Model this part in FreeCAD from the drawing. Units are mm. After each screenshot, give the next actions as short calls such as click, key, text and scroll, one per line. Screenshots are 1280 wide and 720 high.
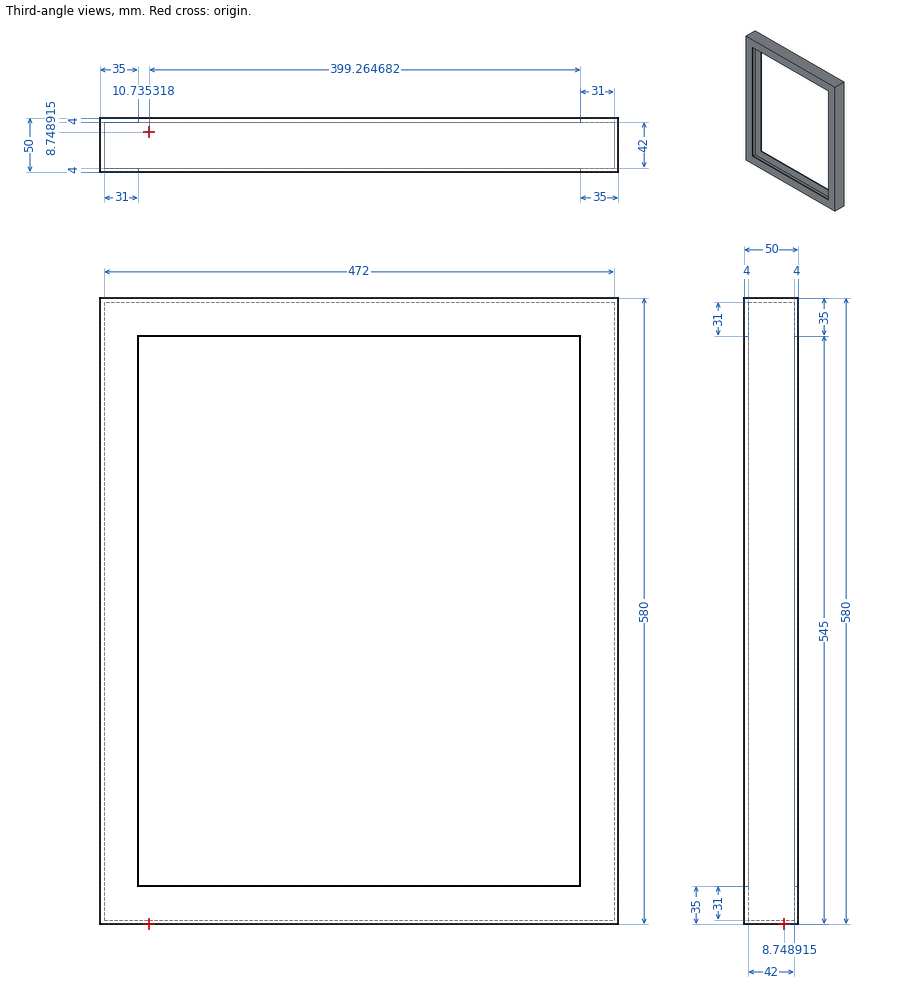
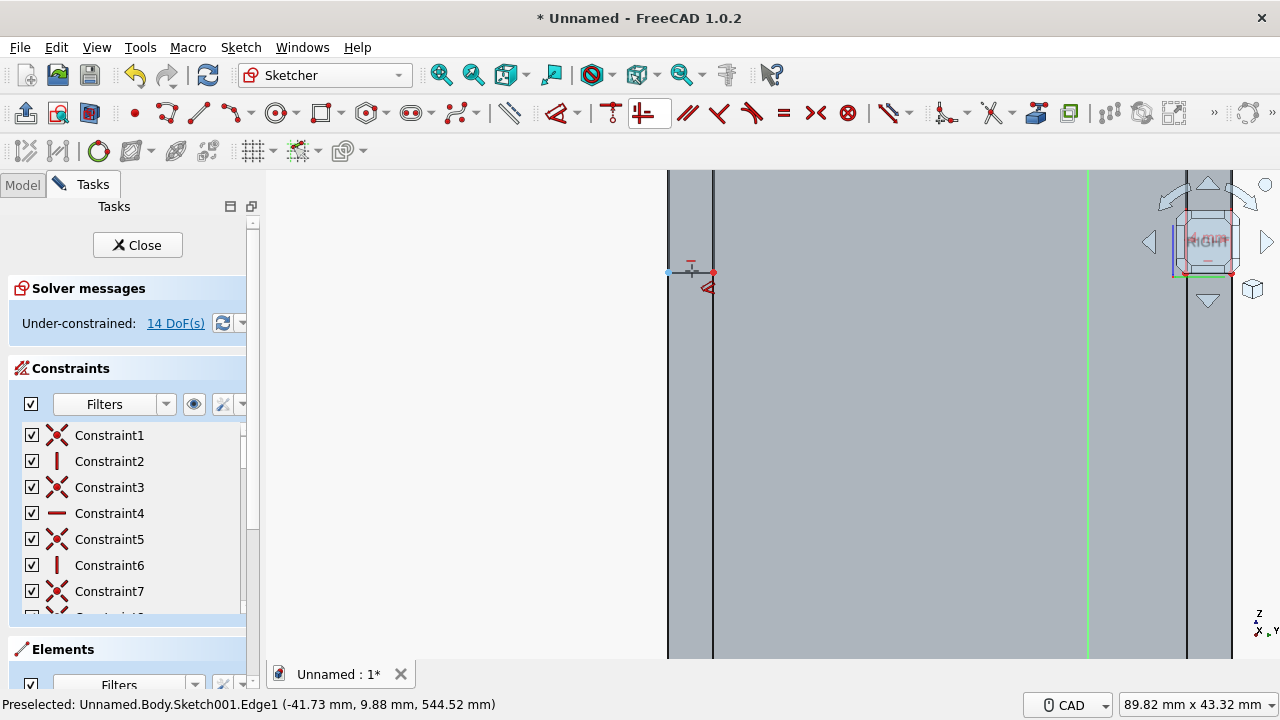
click(682, 273)
click(691, 239)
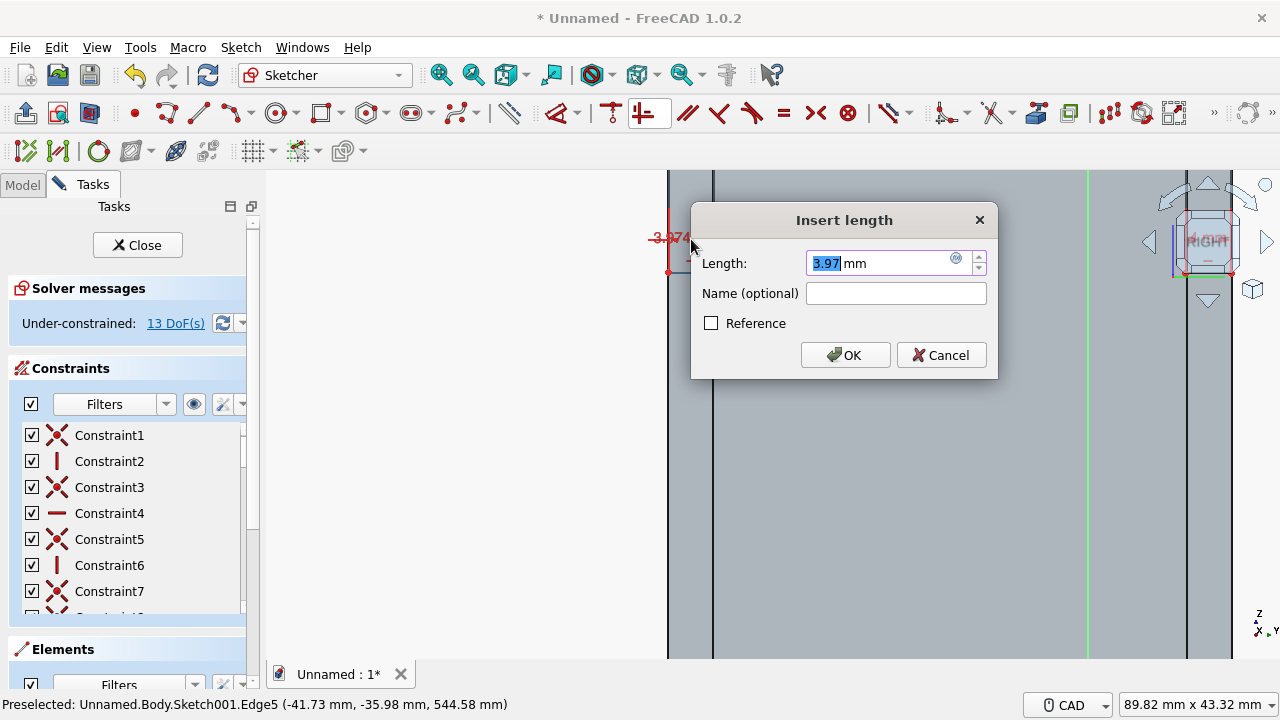
text(4)
key(Return)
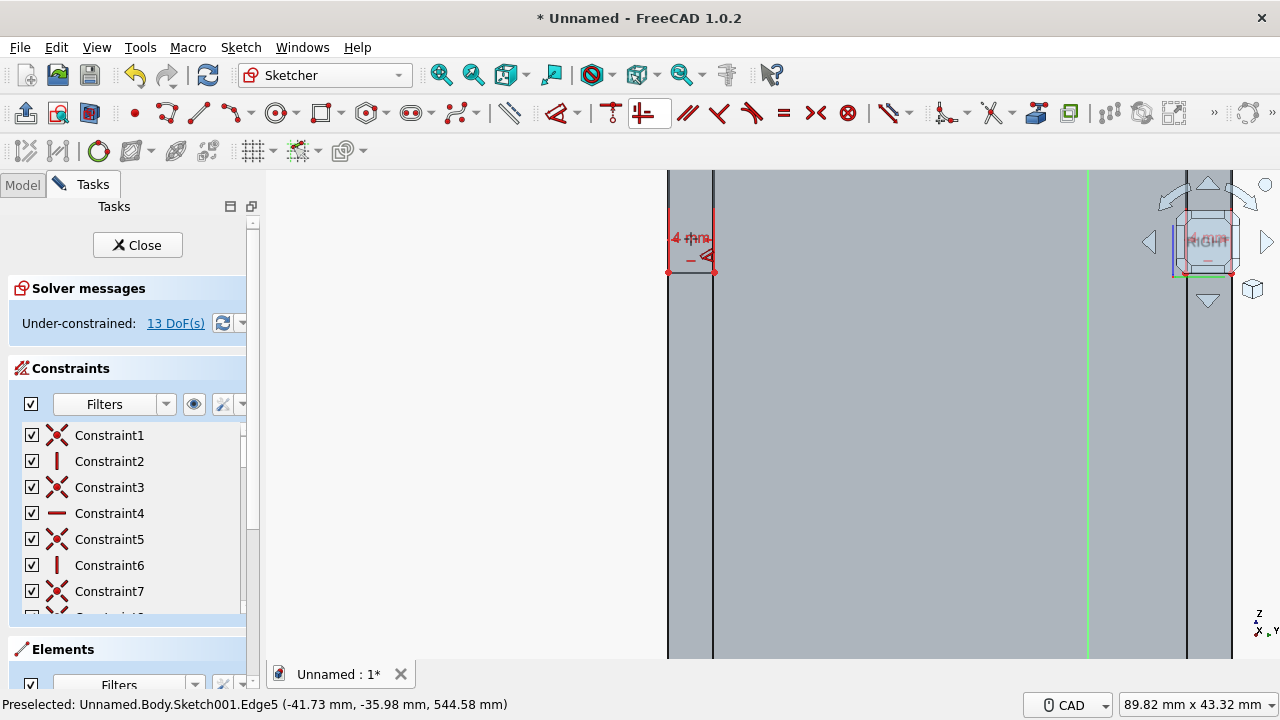
scroll(692, 271, down, 15)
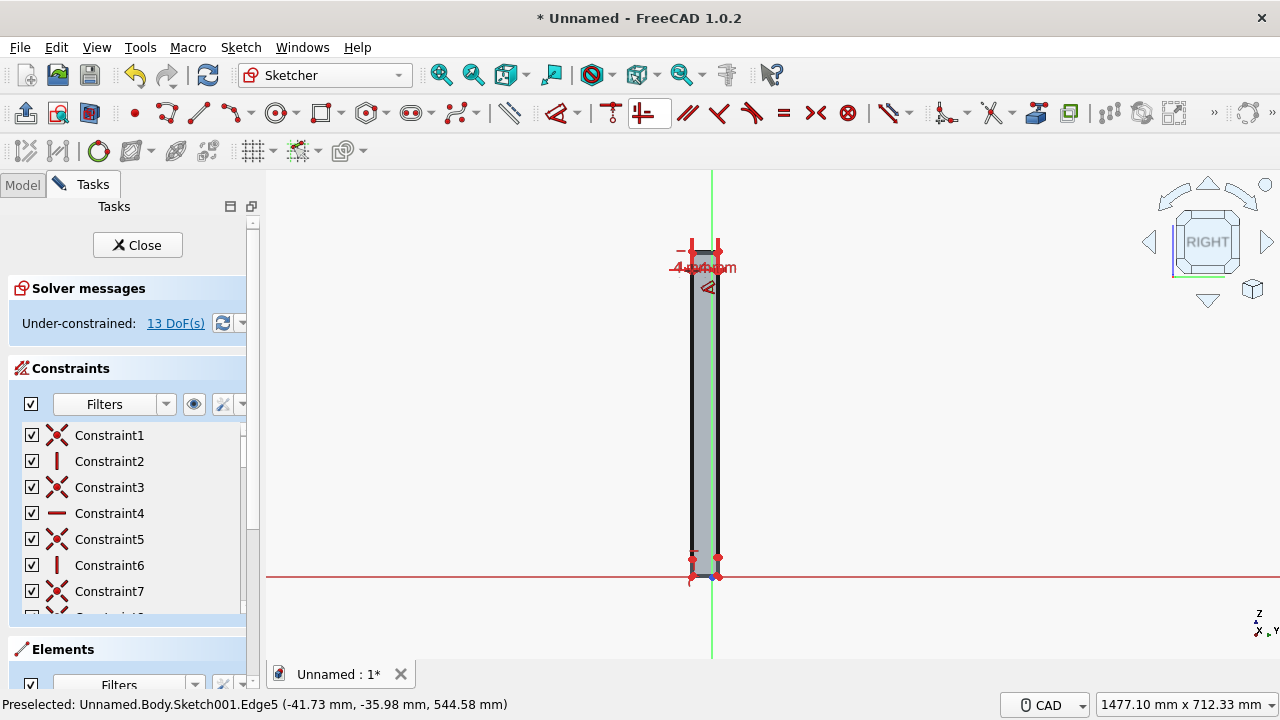
scroll(693, 559, up, 15)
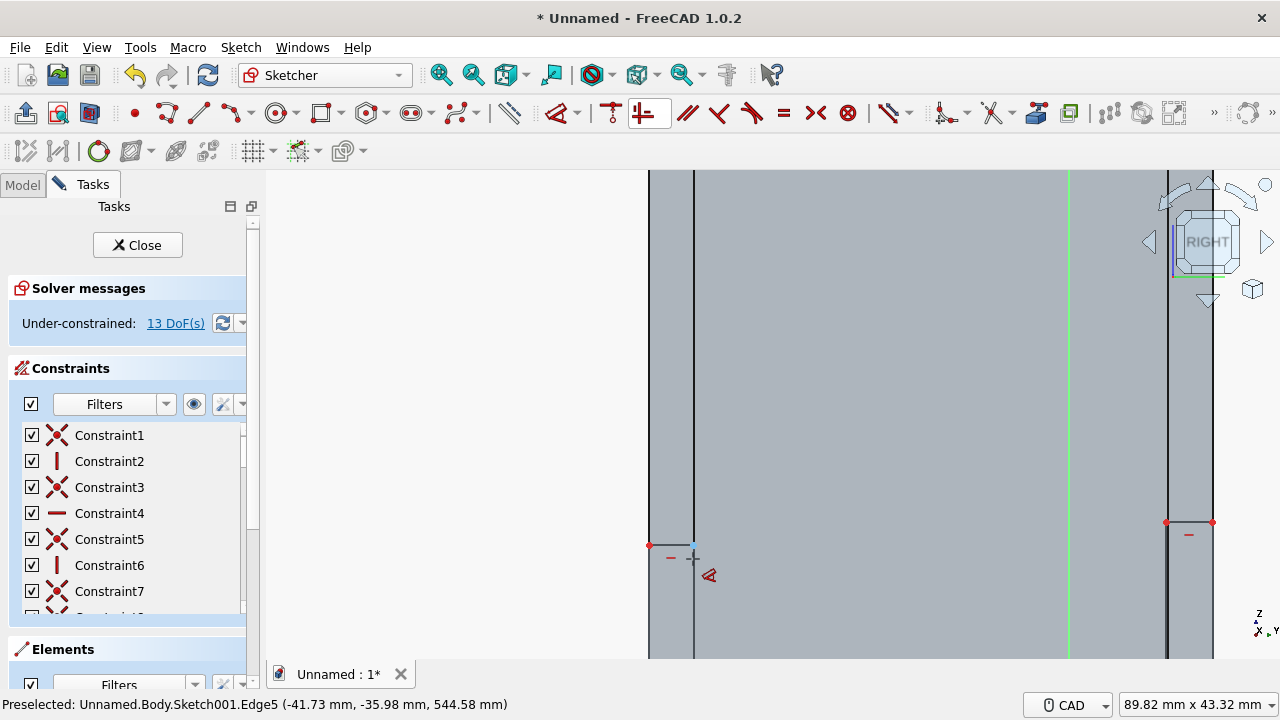
click(680, 545)
click(671, 579)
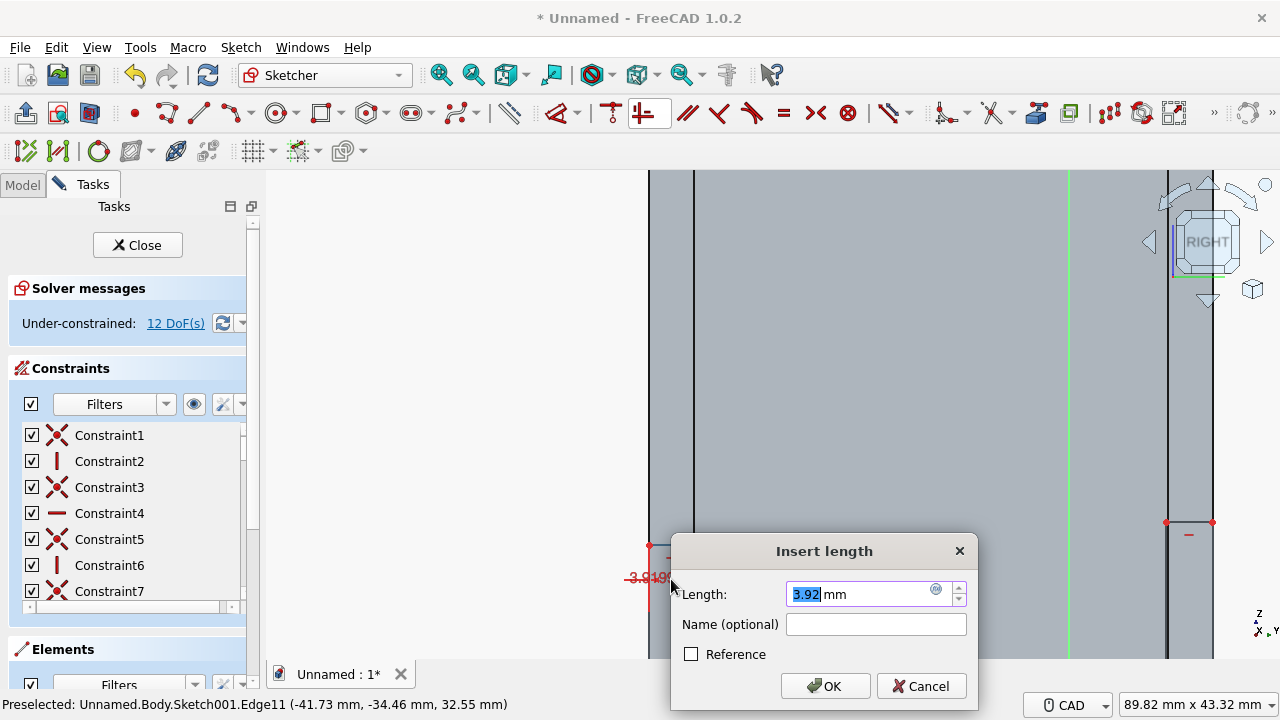
text(4)
key(Return)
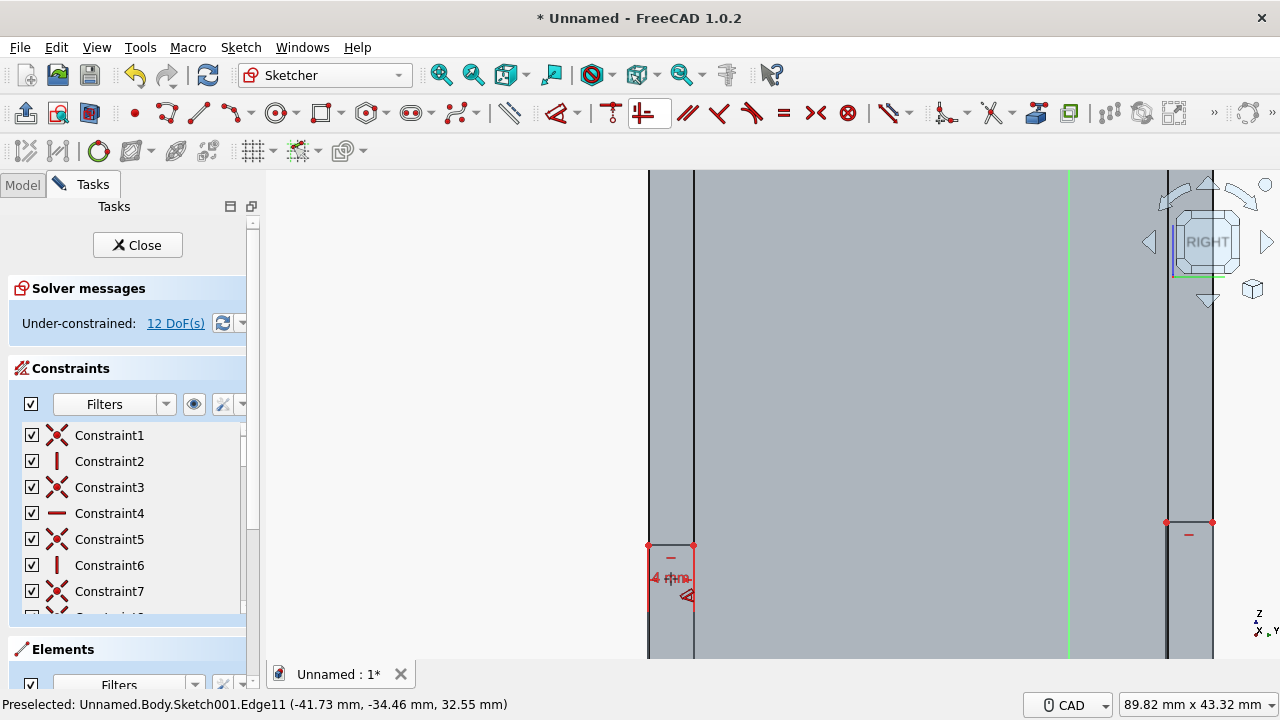
scroll(693, 560, down, 15)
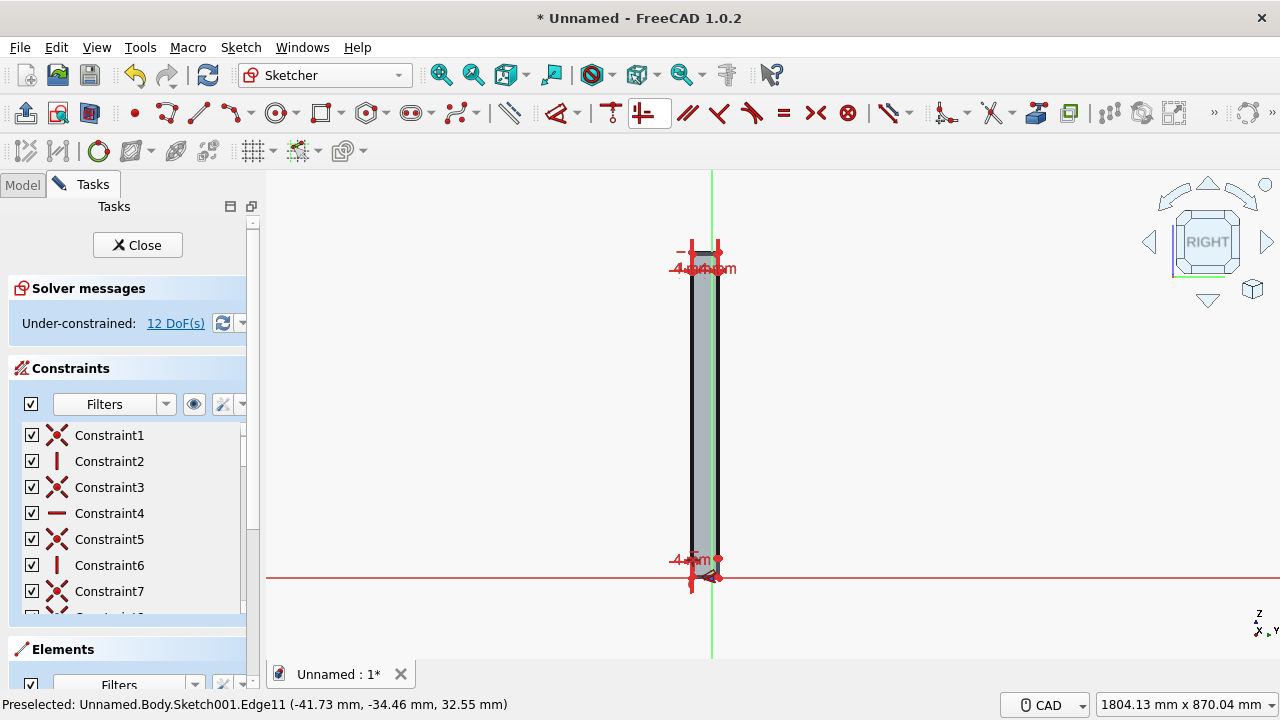
scroll(719, 559, up, 15)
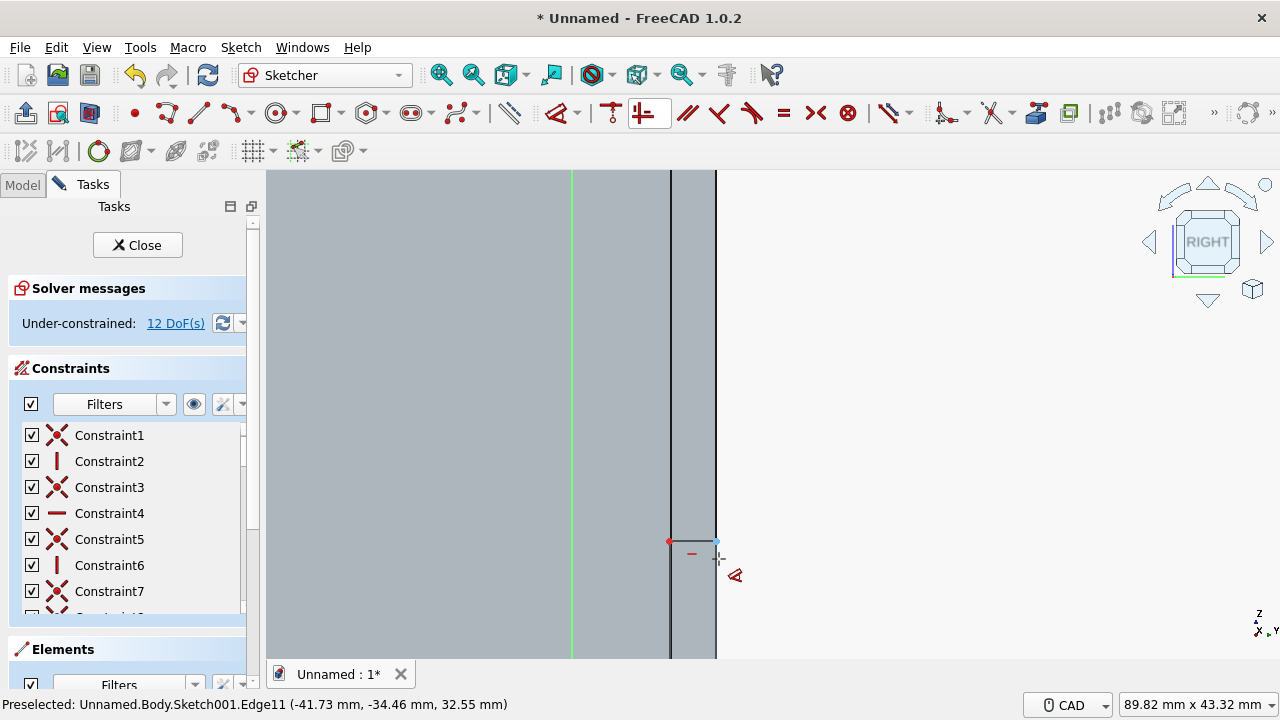
click(702, 541)
click(693, 575)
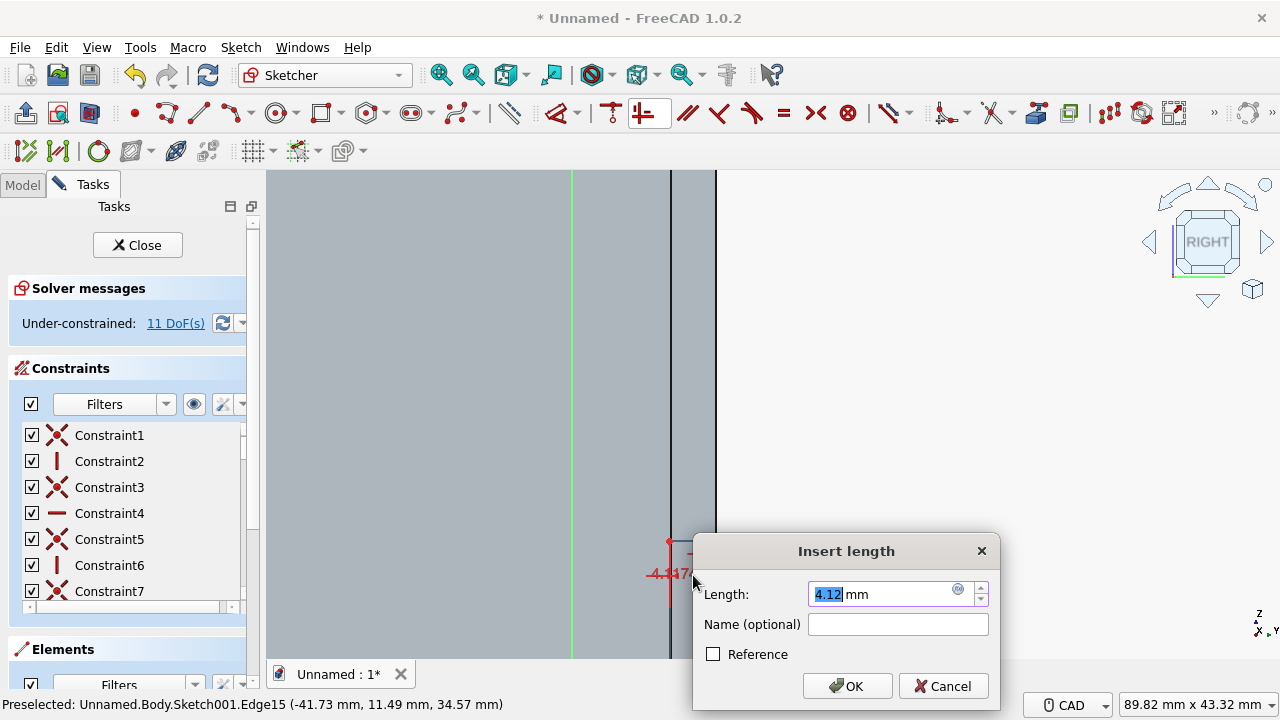
text(4)
key(Return)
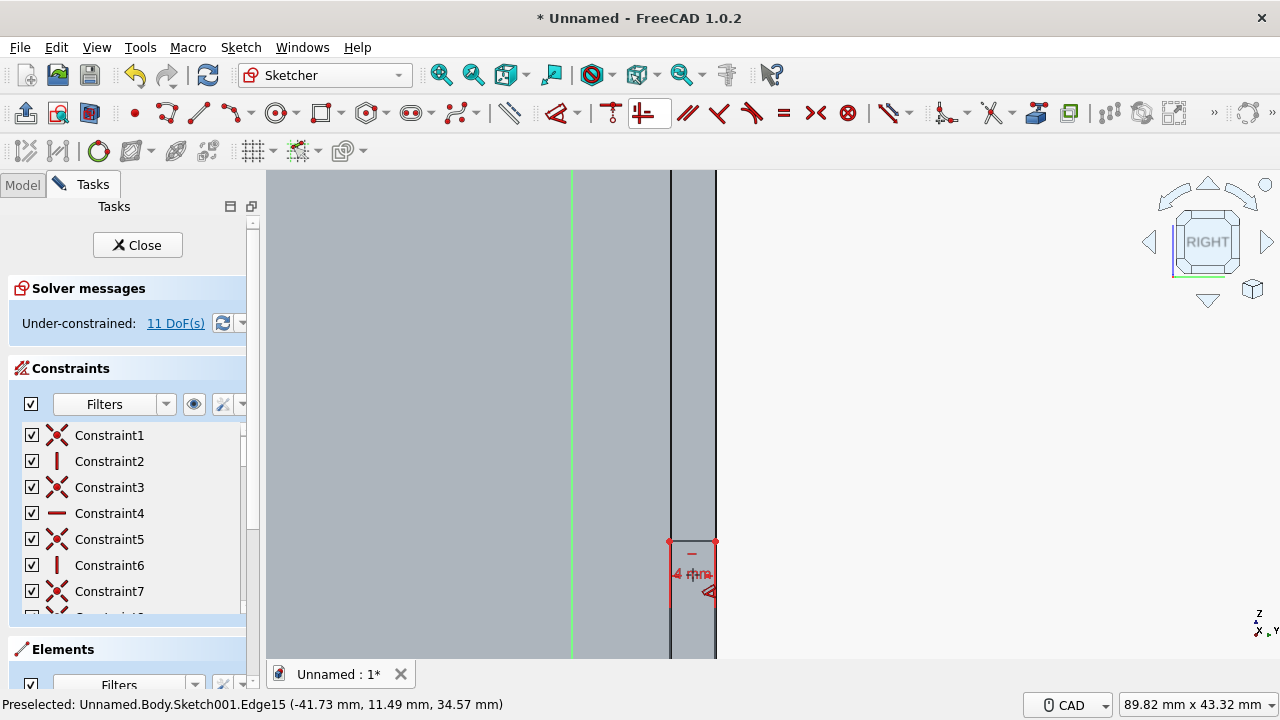
scroll(719, 559, down, 15)